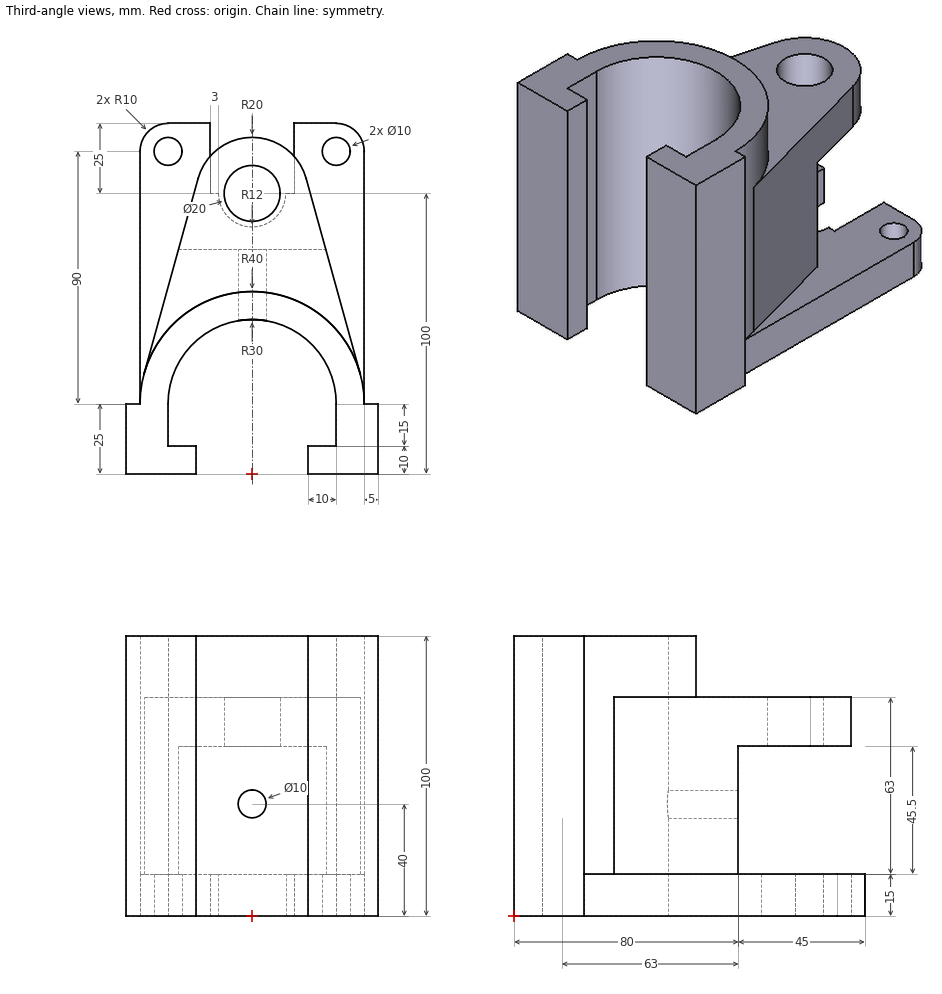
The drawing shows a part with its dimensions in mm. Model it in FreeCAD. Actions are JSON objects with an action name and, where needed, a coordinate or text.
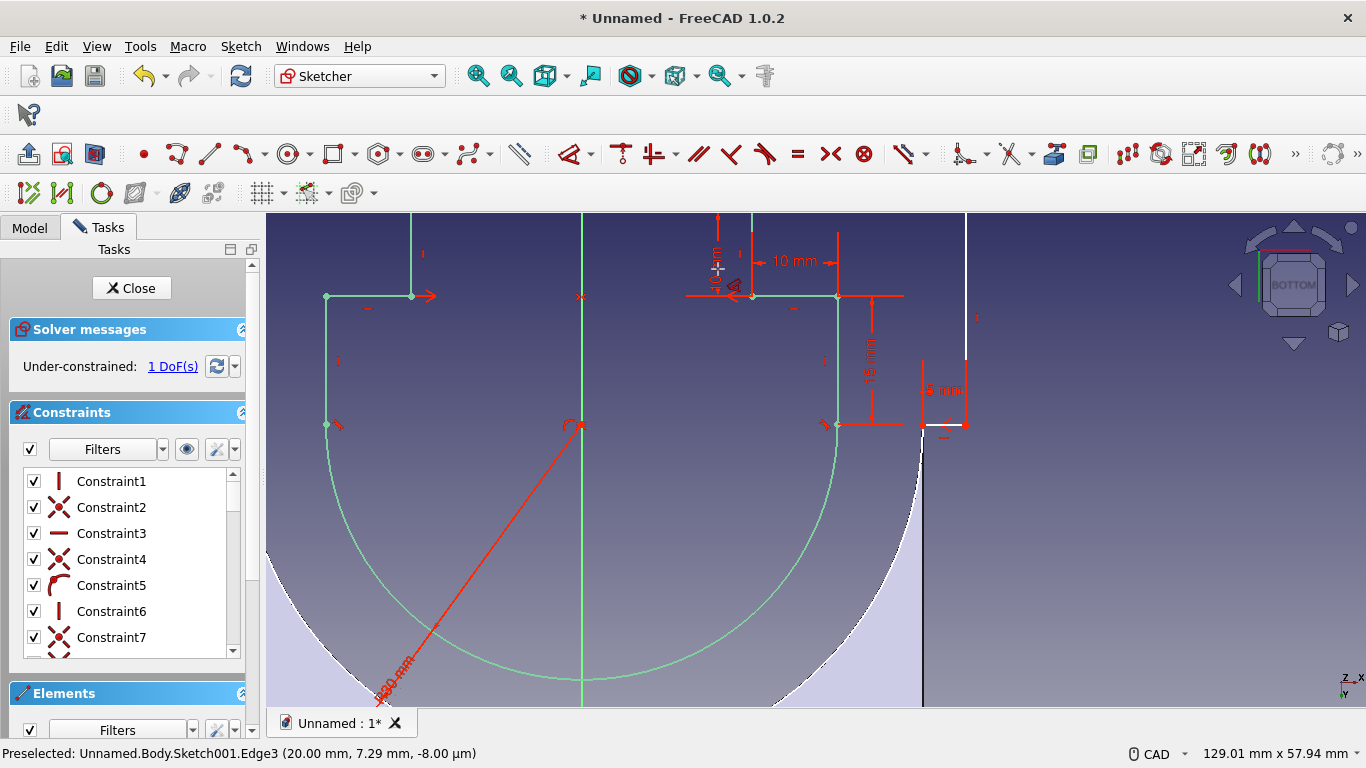
{"action": "left_click", "coordinate": [966, 275]}
{"action": "left_click", "coordinate": [1000, 333]}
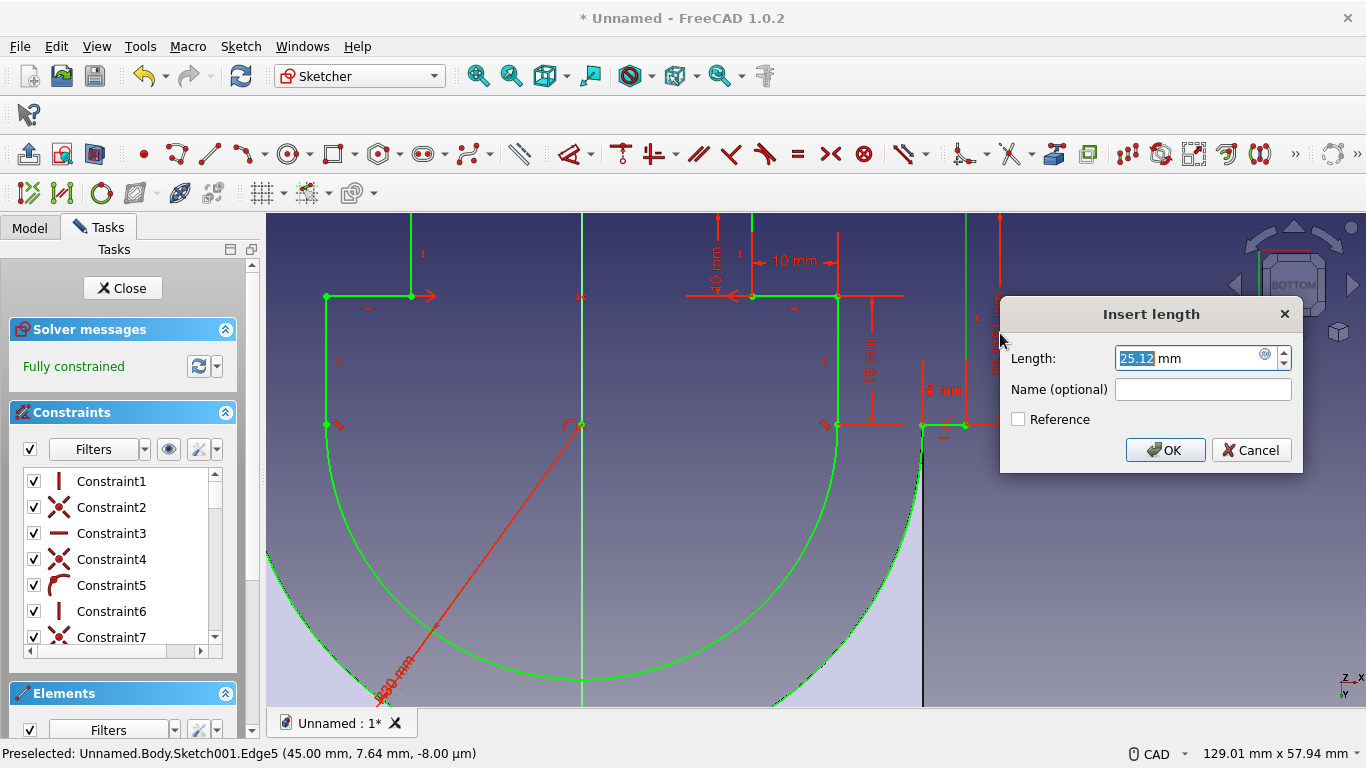
{"action": "type", "text": "25"}
{"action": "key", "text": "Return"}
{"action": "key", "text": "Escape"}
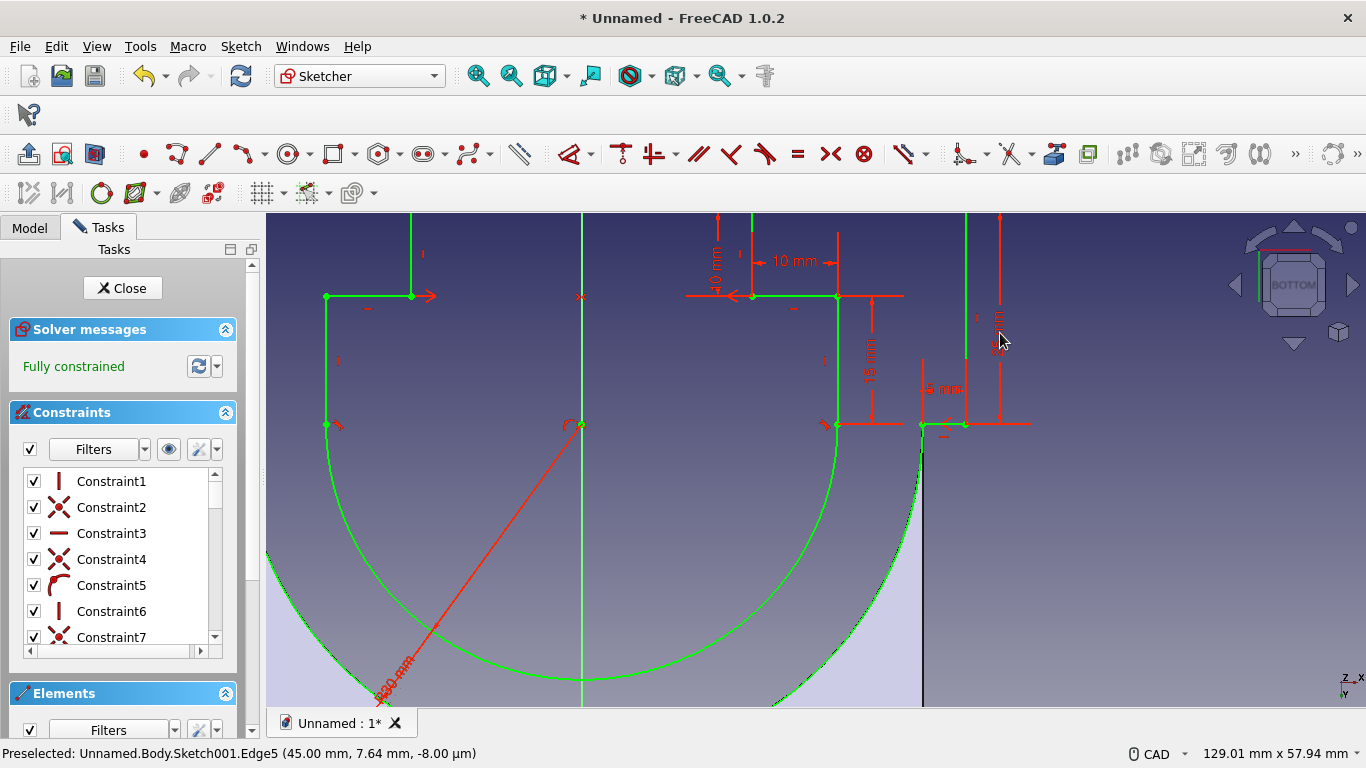
{"action": "left_click", "coordinate": [123, 288]}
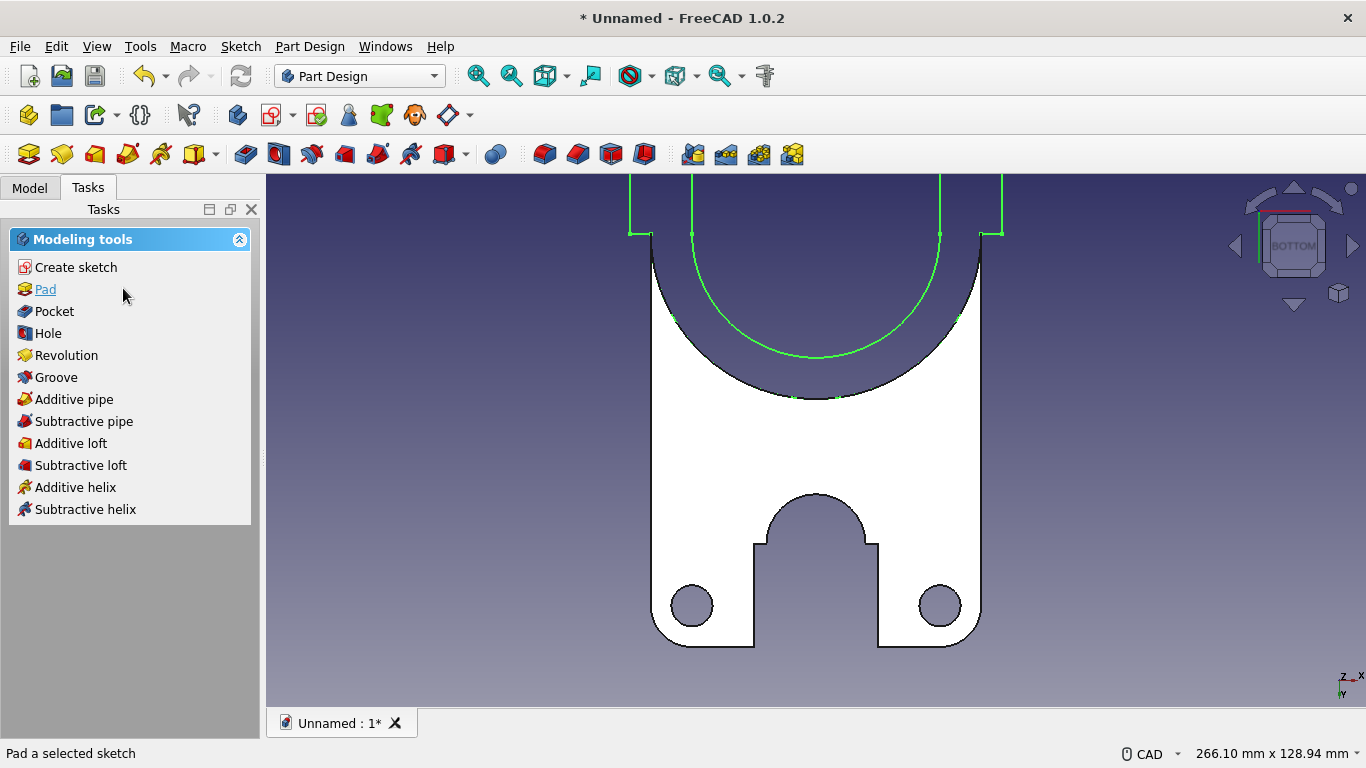
{"action": "left_click", "coordinate": [29, 154]}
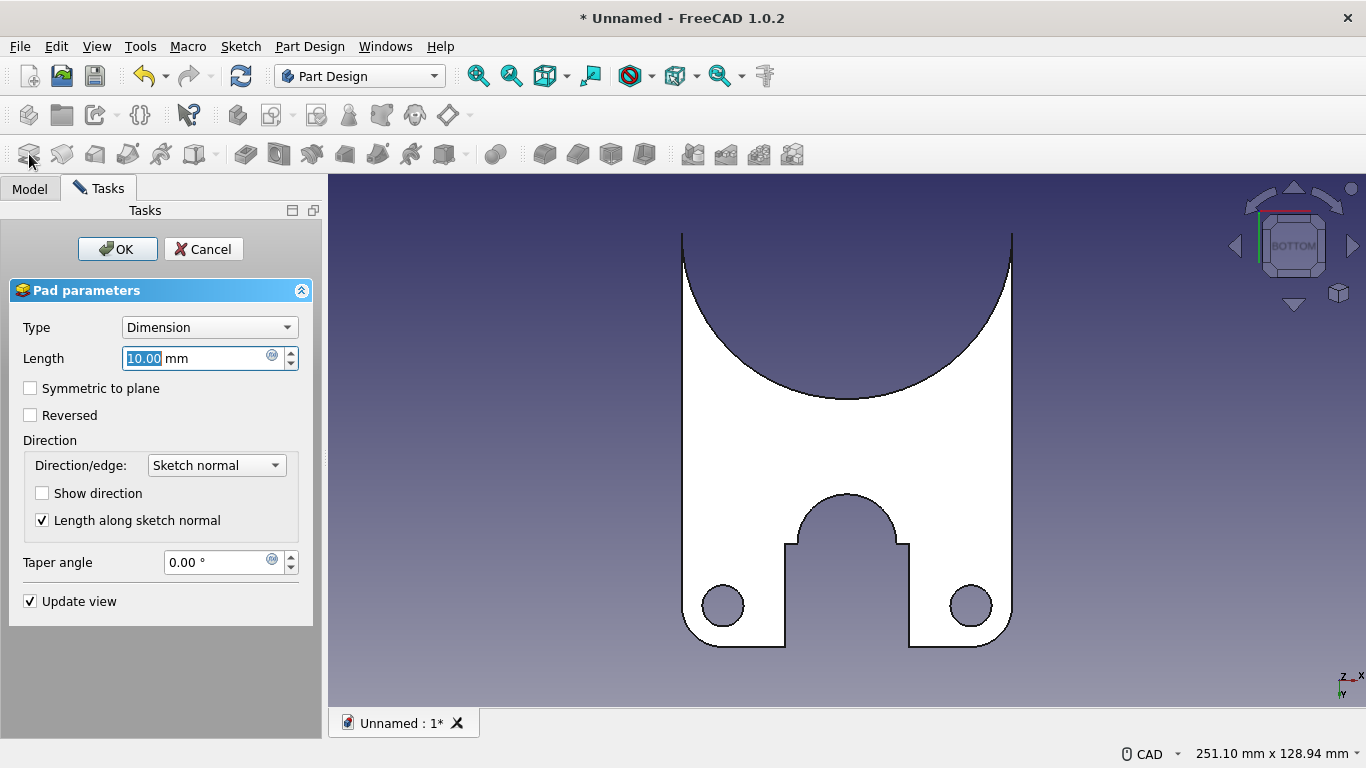
{"action": "type", "text": "100"}
{"action": "key", "text": "Tab"}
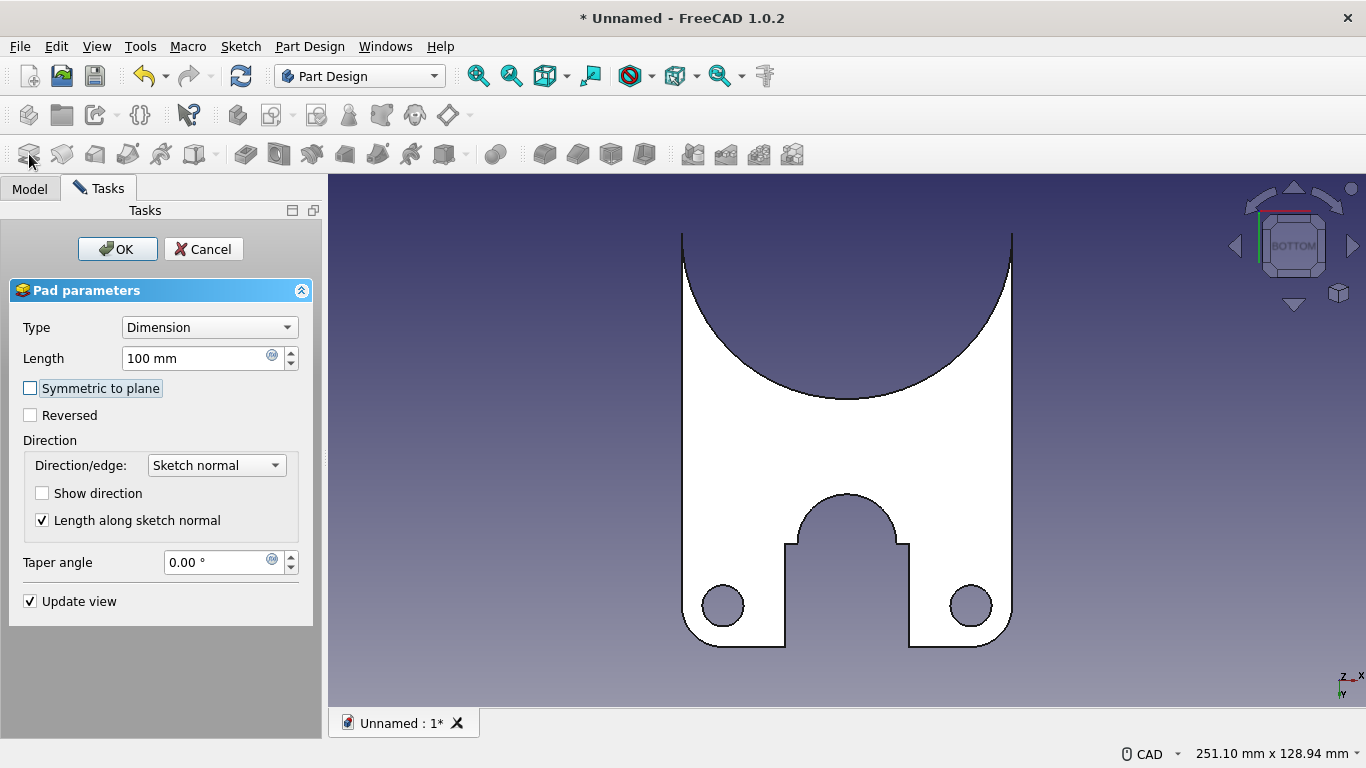
{"action": "left_click", "coordinate": [31, 415]}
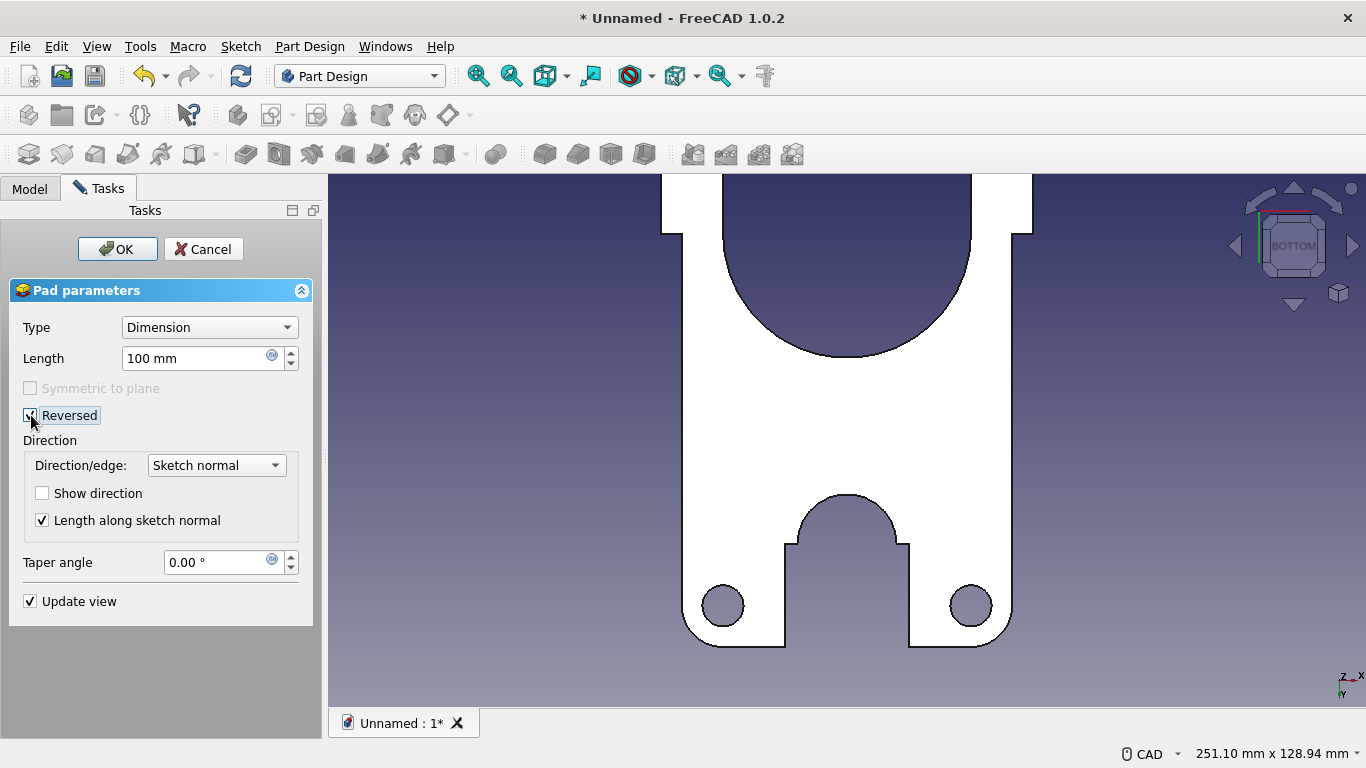
{"action": "left_click", "coordinate": [118, 249]}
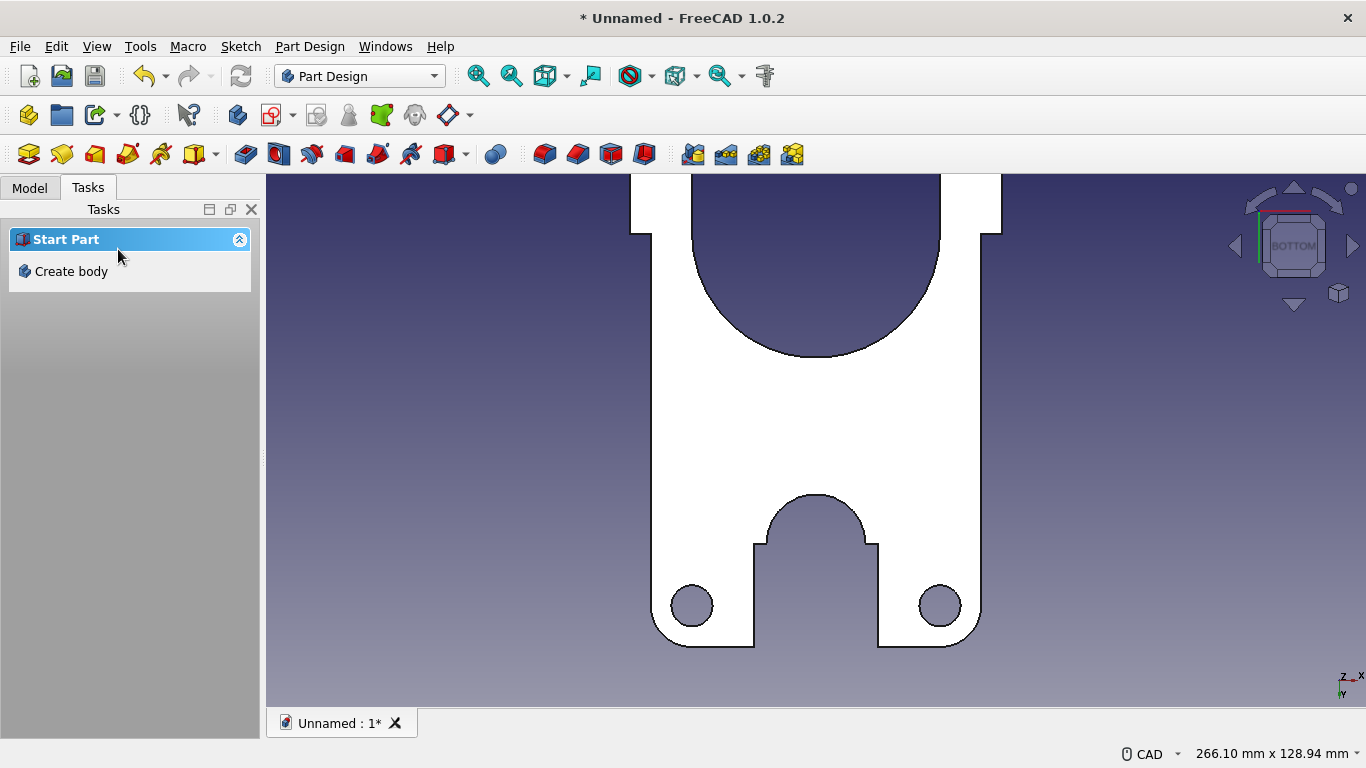
{"action": "key", "text": "v f"}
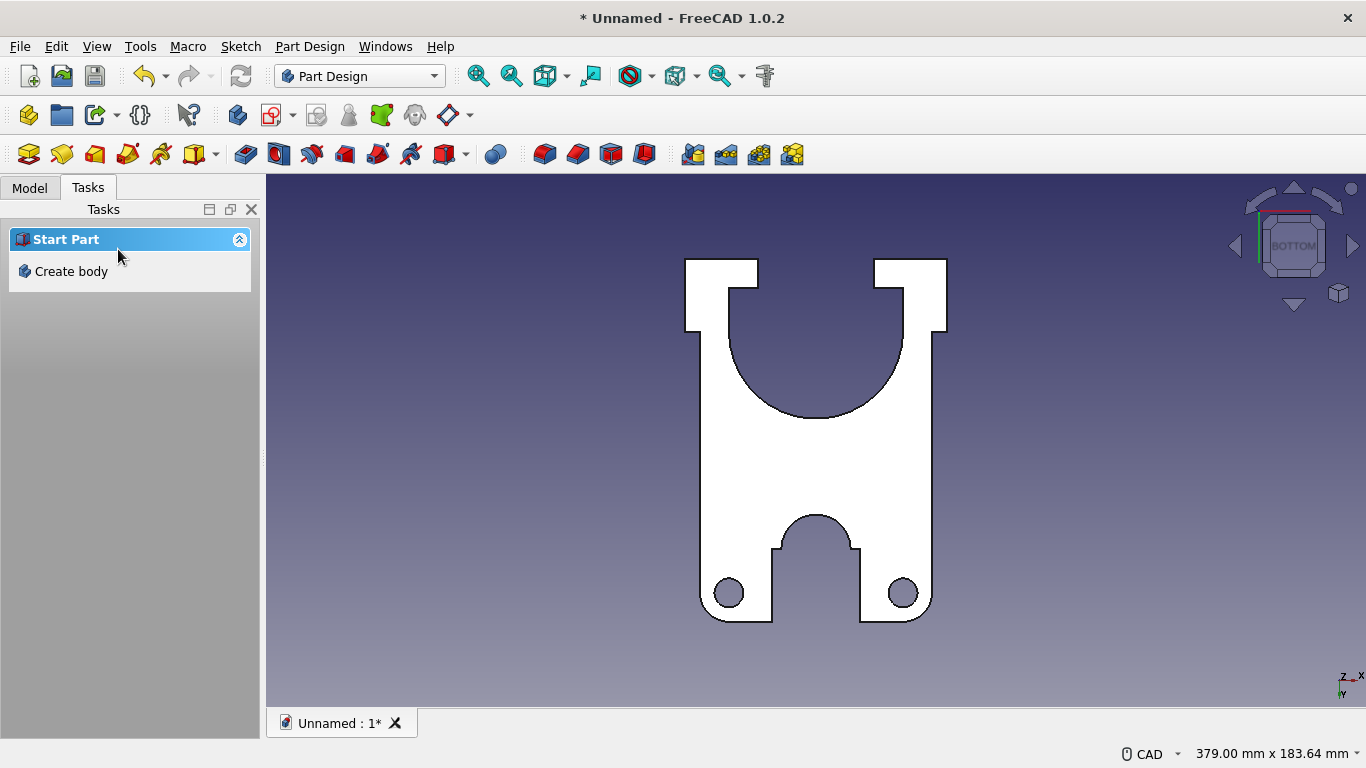
{"action": "key", "text": "0"}